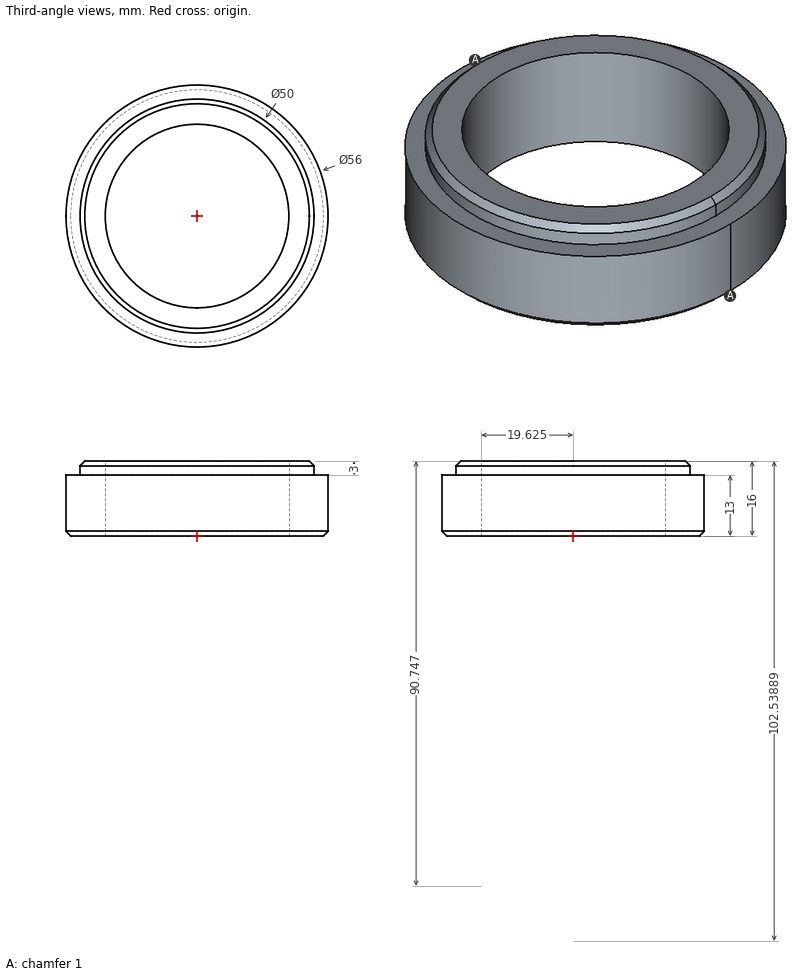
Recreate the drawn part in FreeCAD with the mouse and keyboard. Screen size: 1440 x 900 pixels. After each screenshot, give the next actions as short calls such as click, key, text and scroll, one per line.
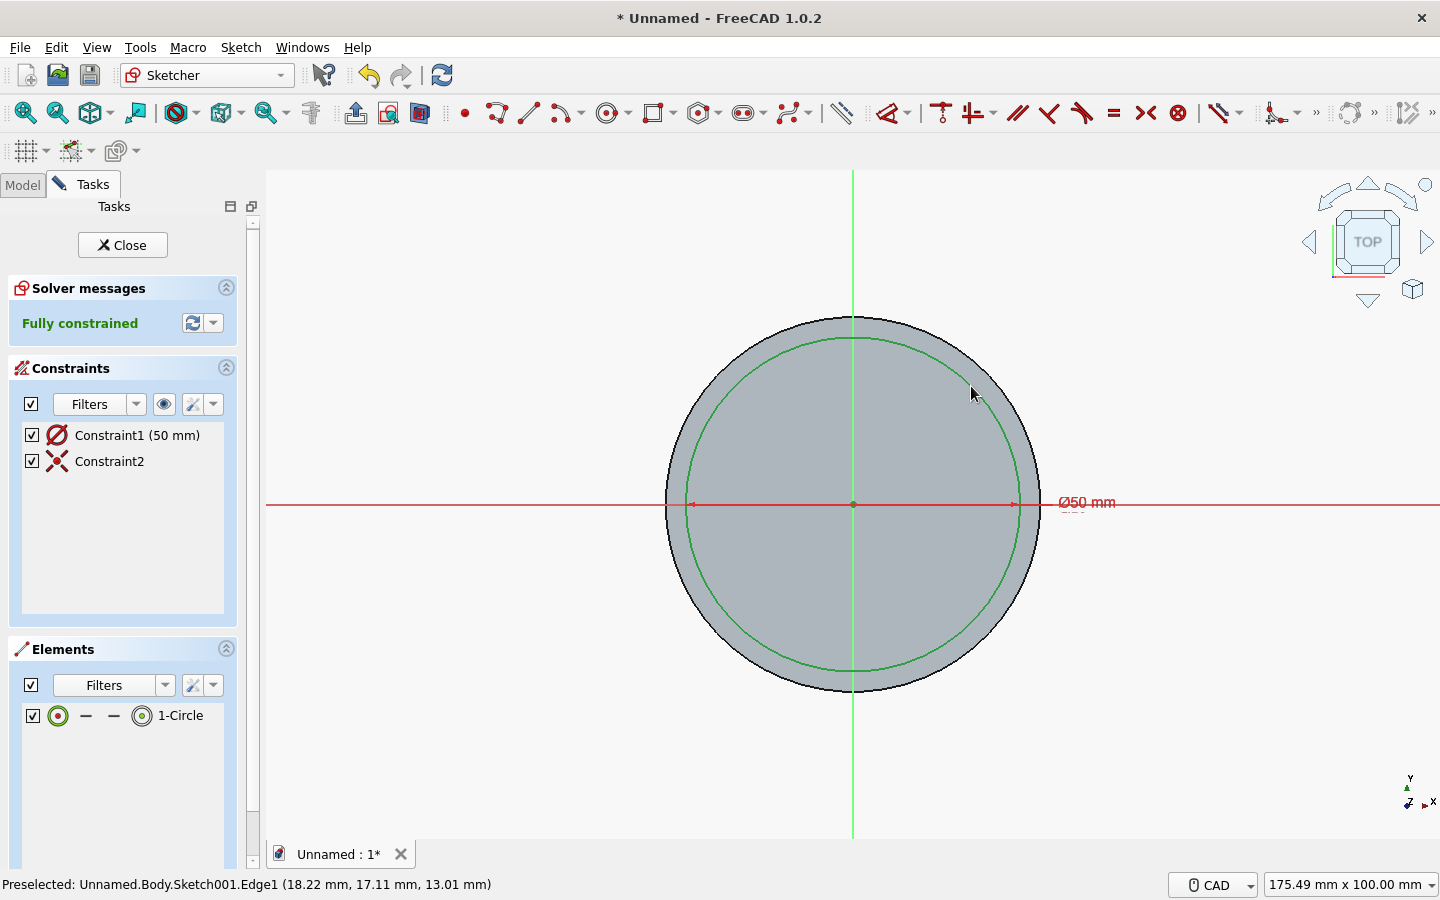
click(123, 245)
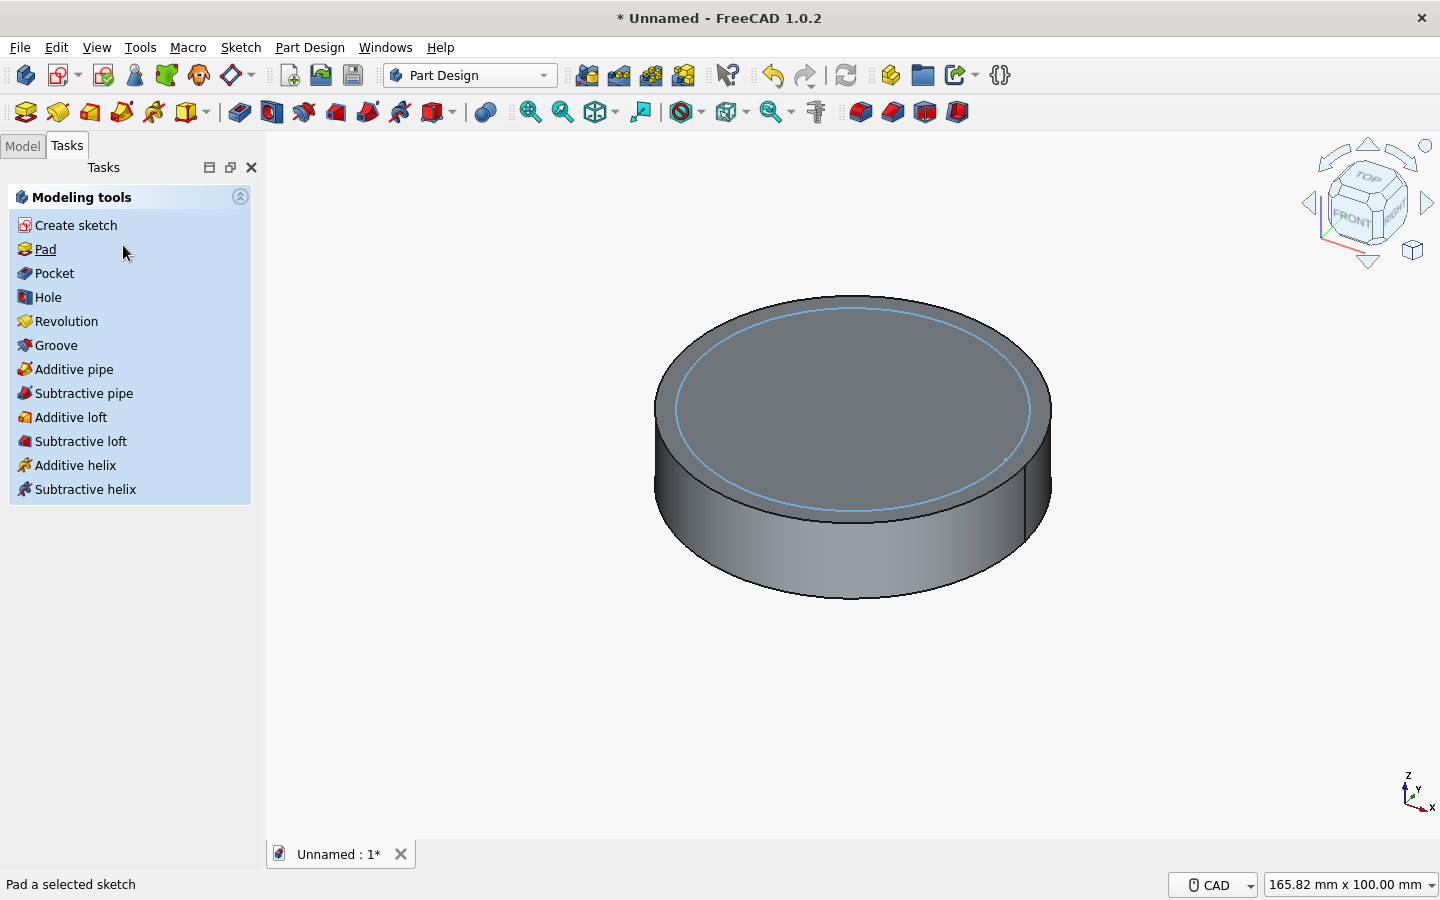
click(26, 112)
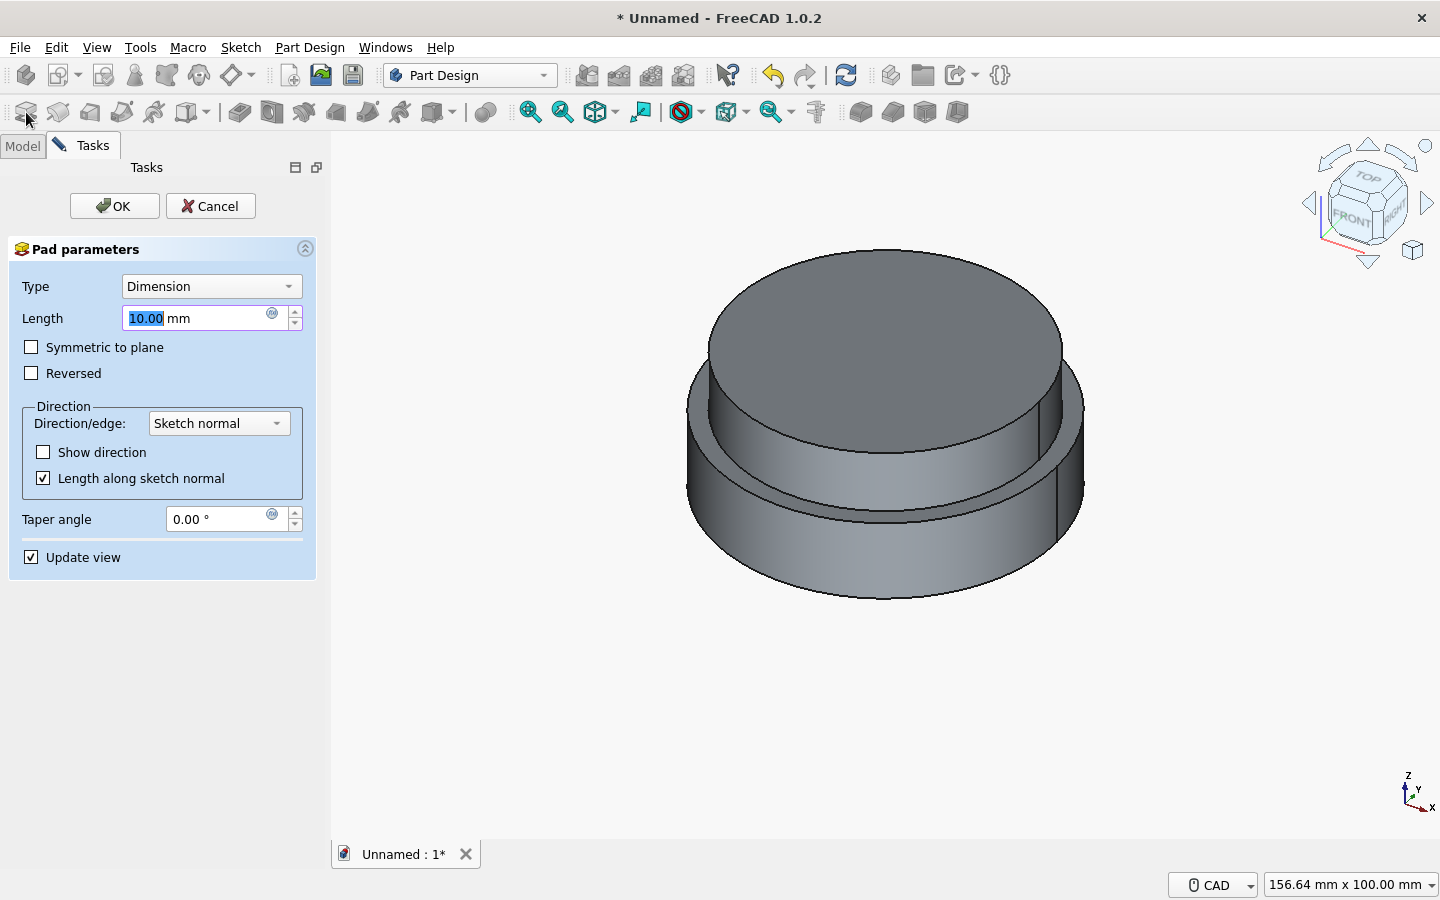
text(3)
key(Tab)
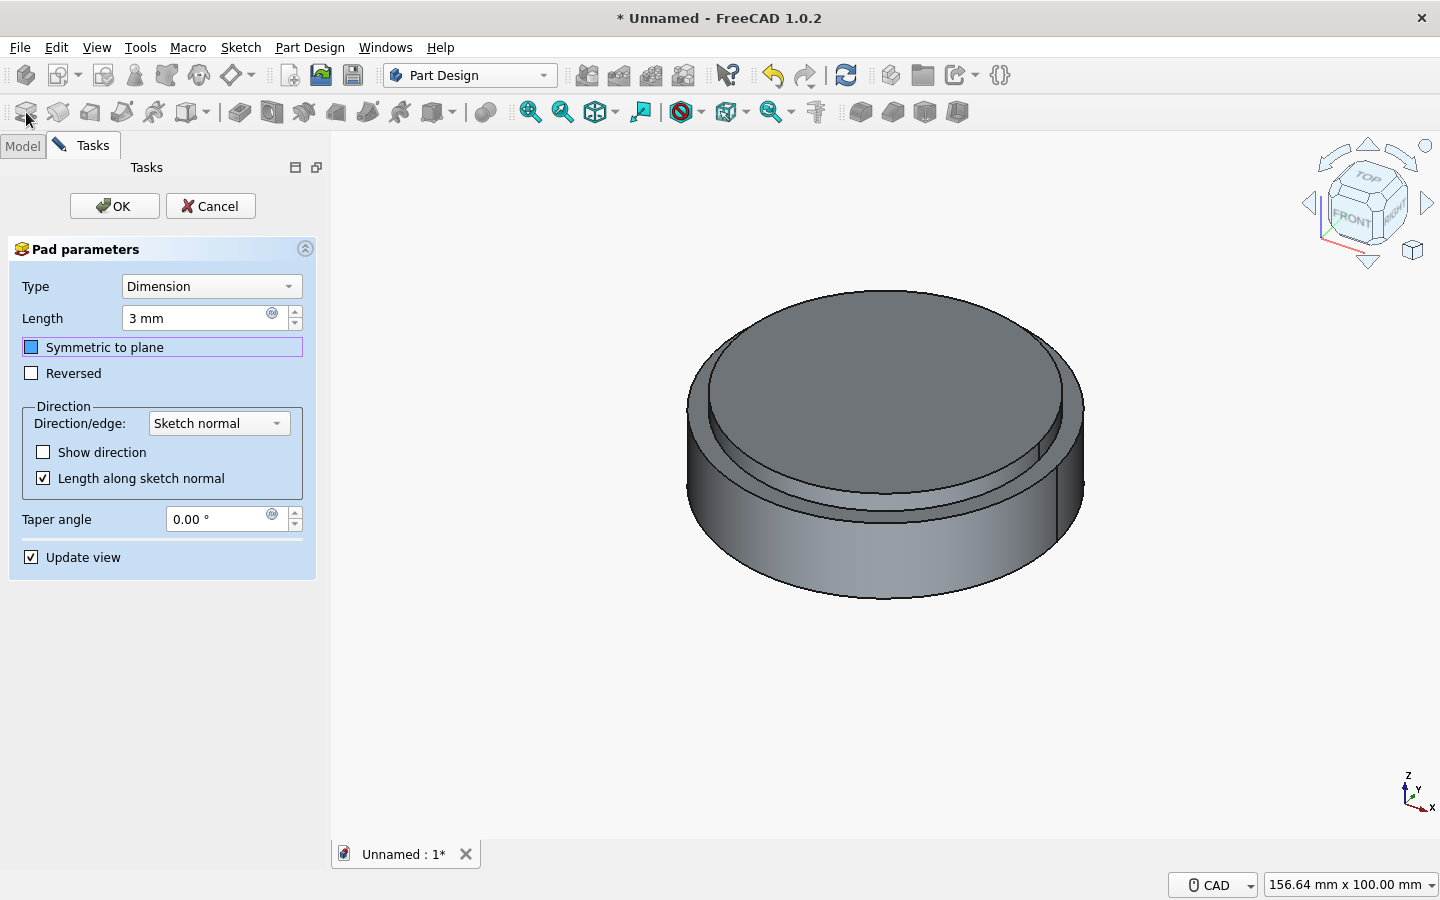
click(115, 206)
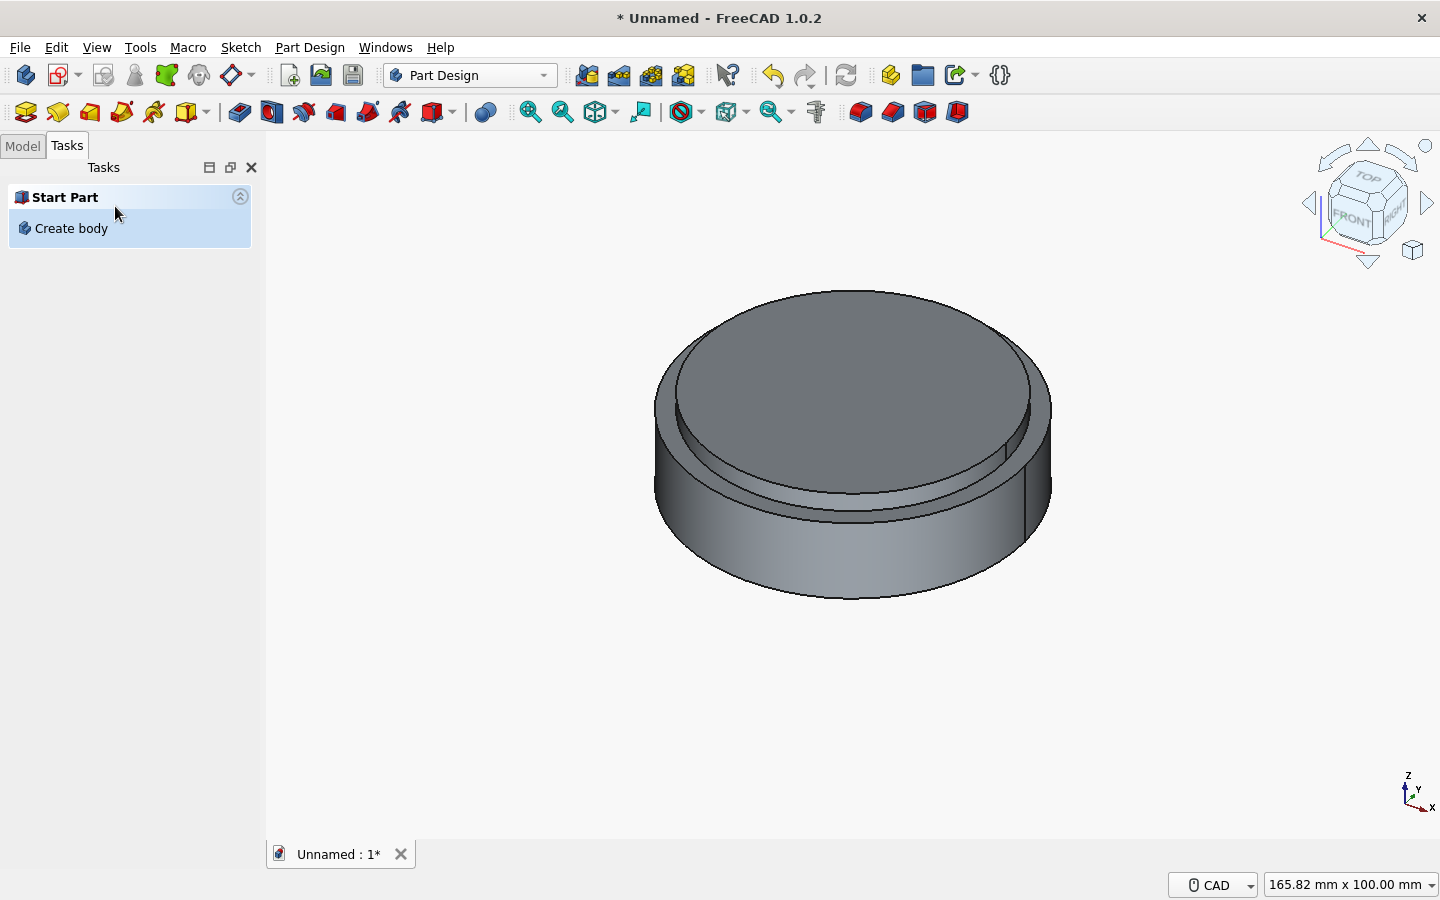
click(677, 402)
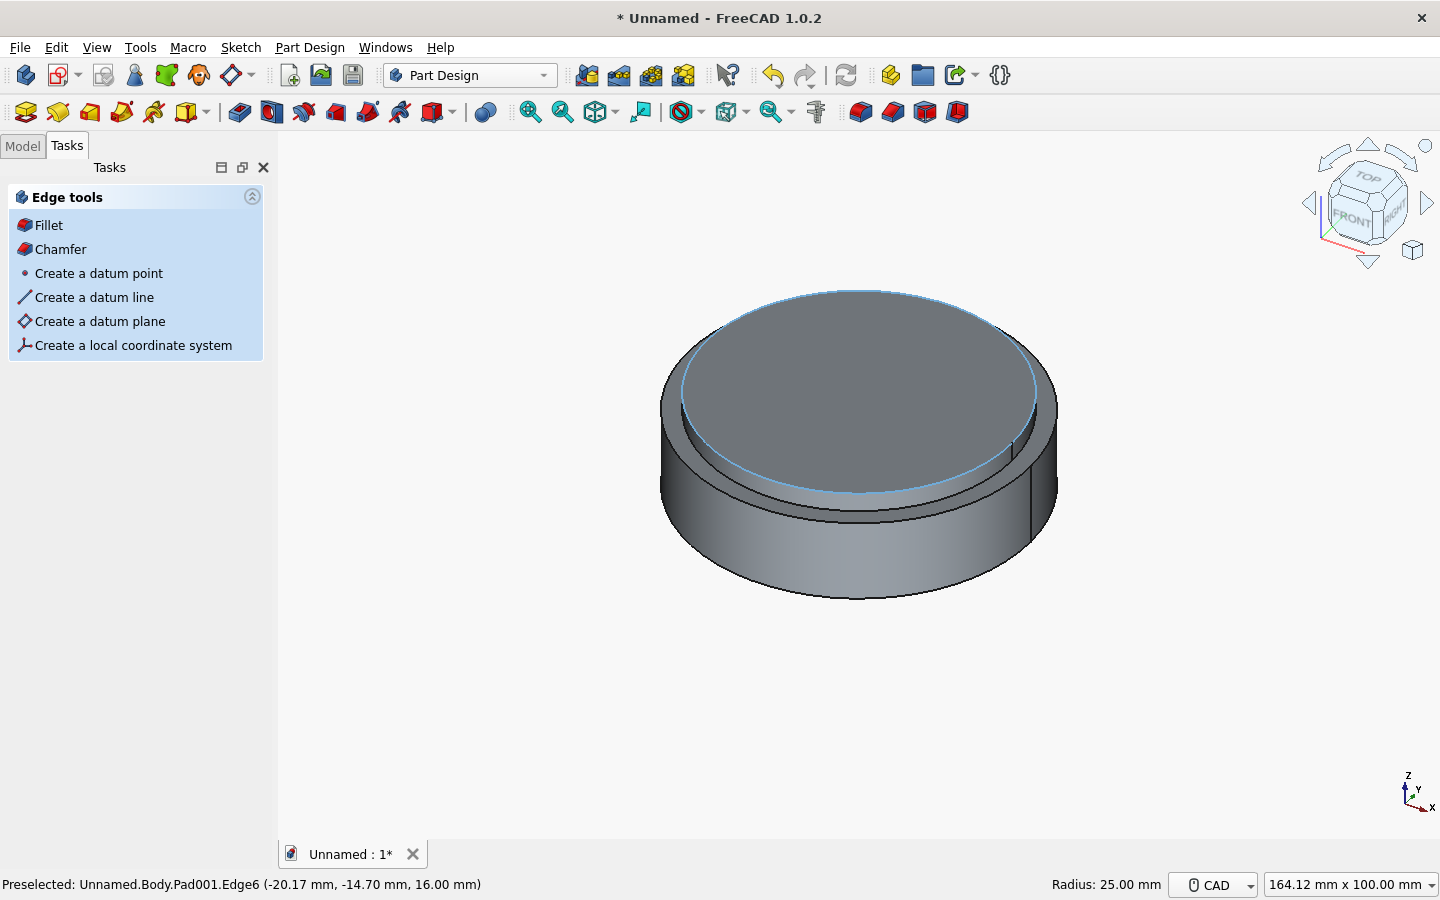
key(0)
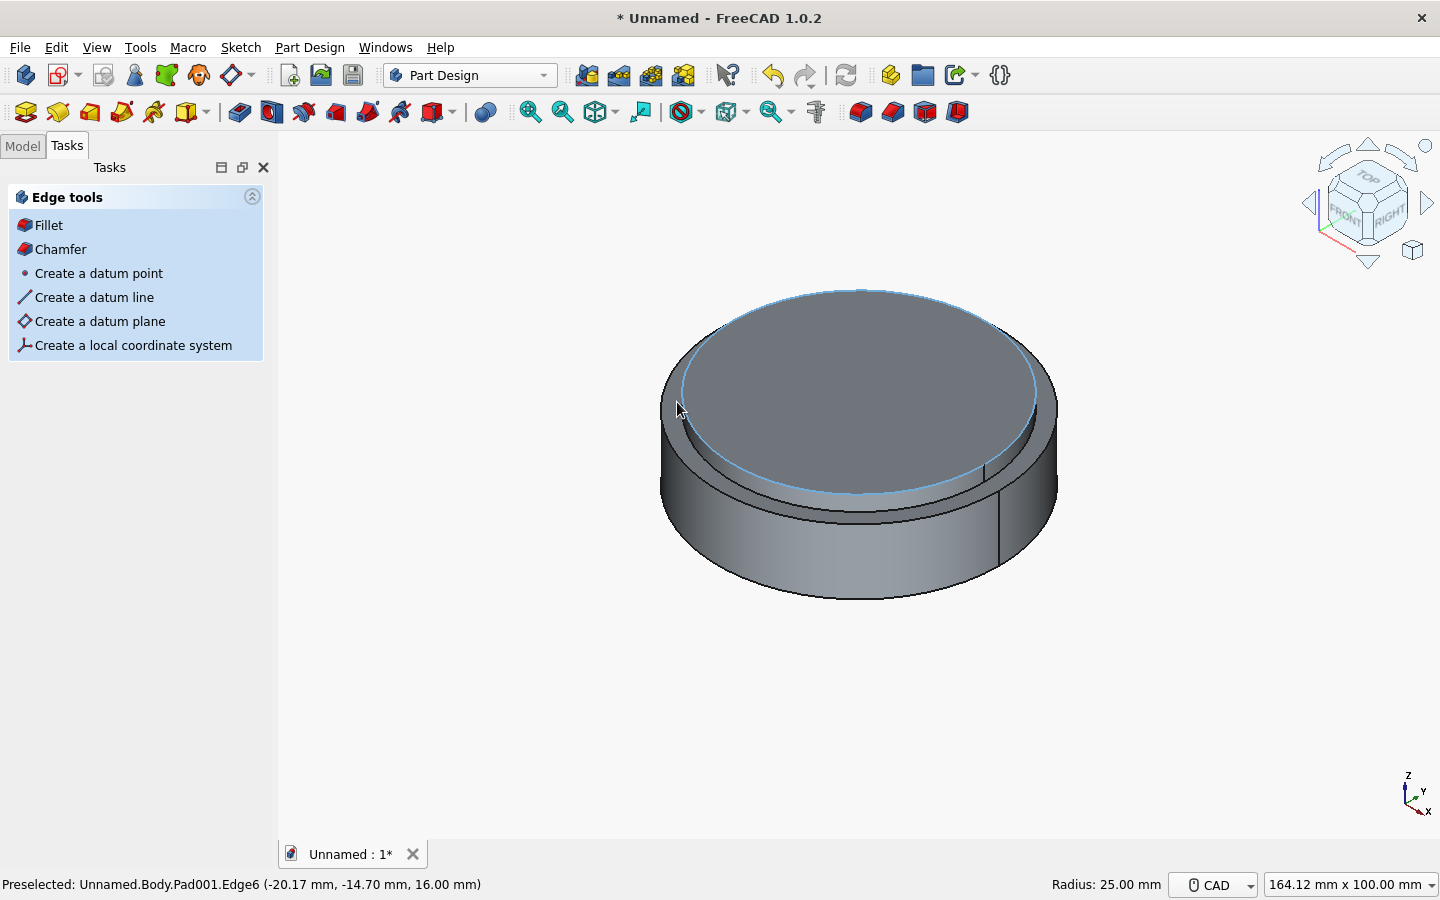
key(2)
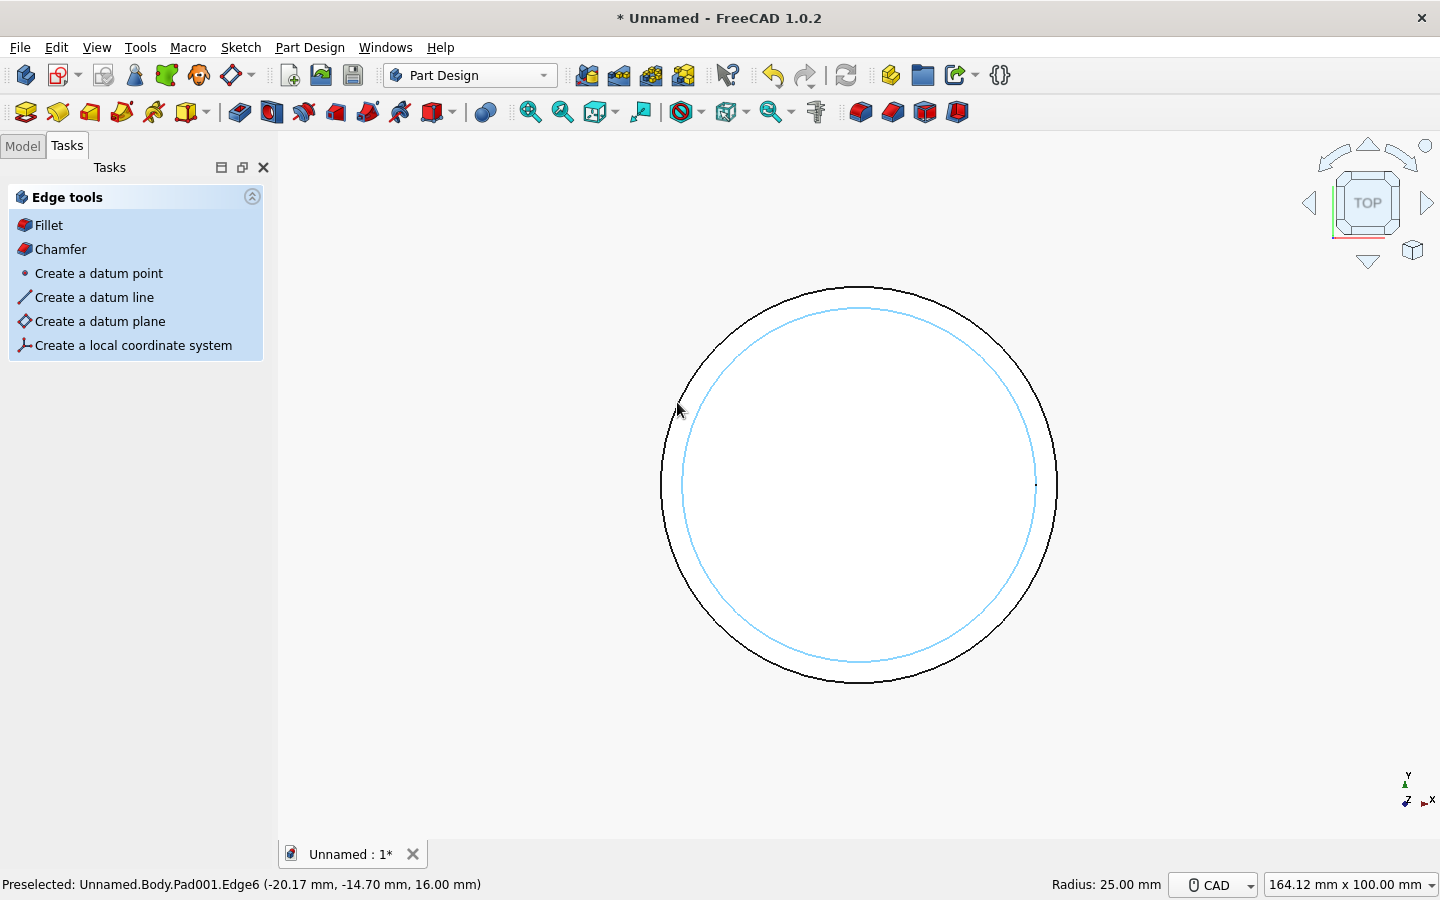
key(1)